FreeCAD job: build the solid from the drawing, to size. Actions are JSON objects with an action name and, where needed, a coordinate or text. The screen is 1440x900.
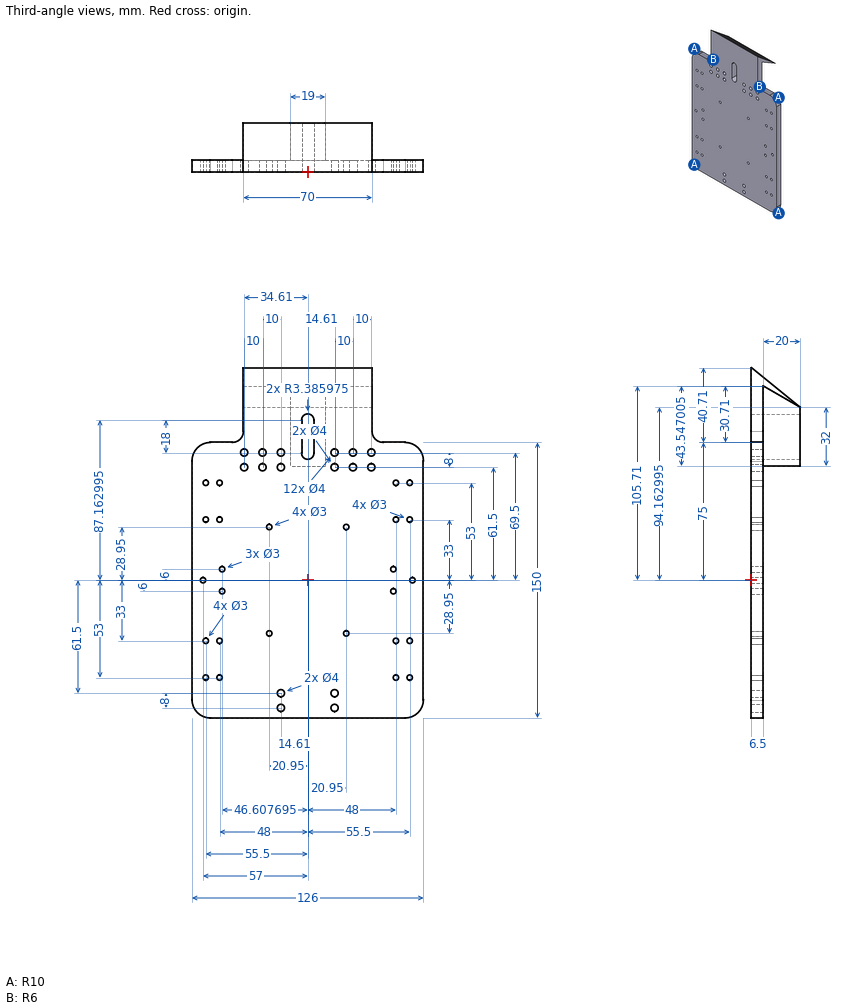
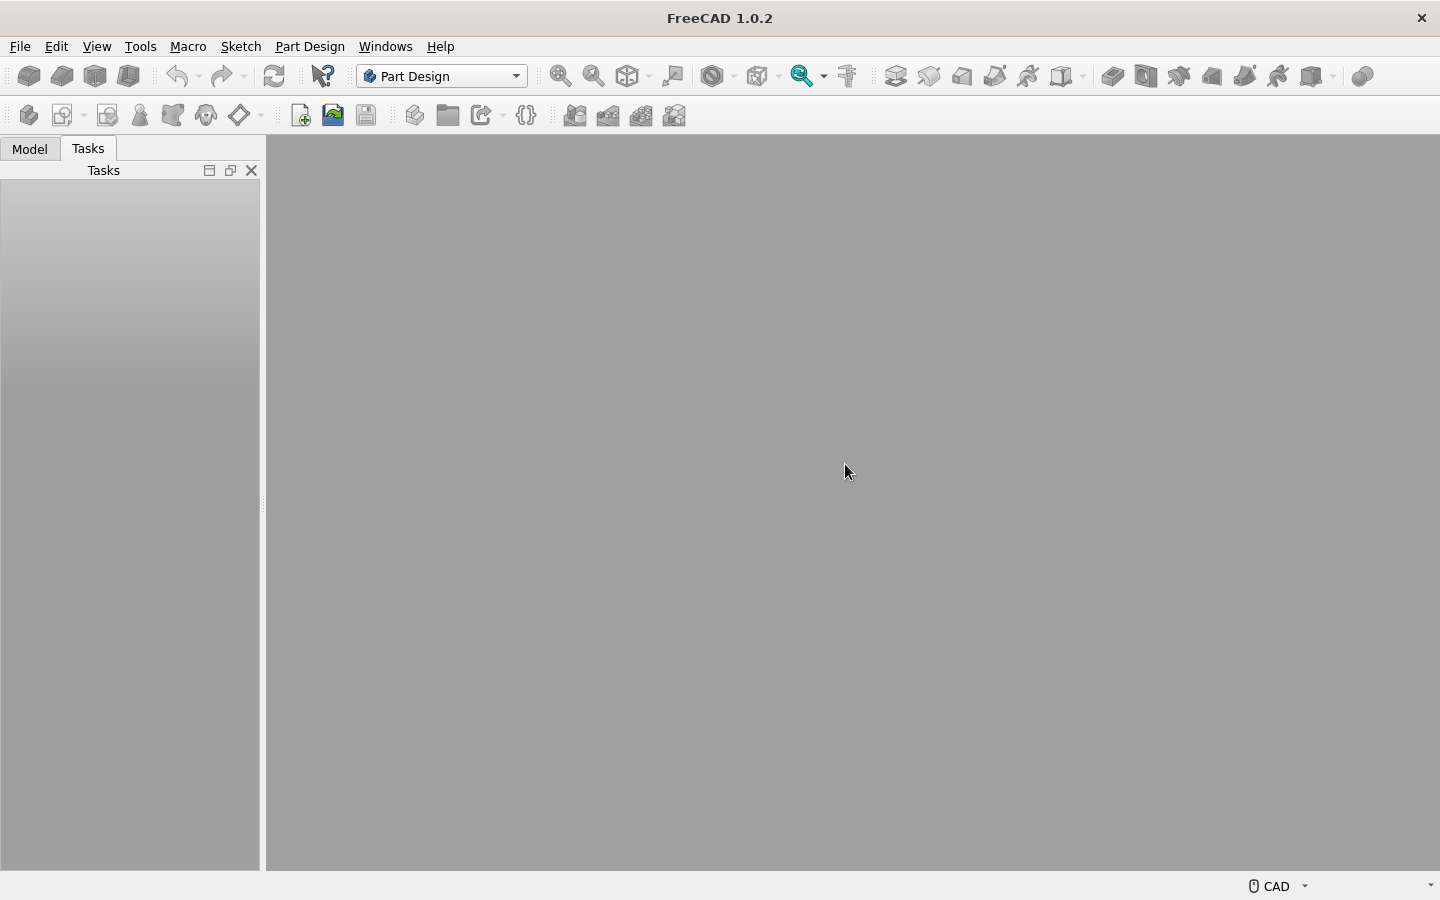
{"action": "left_click", "coordinate": [300, 116]}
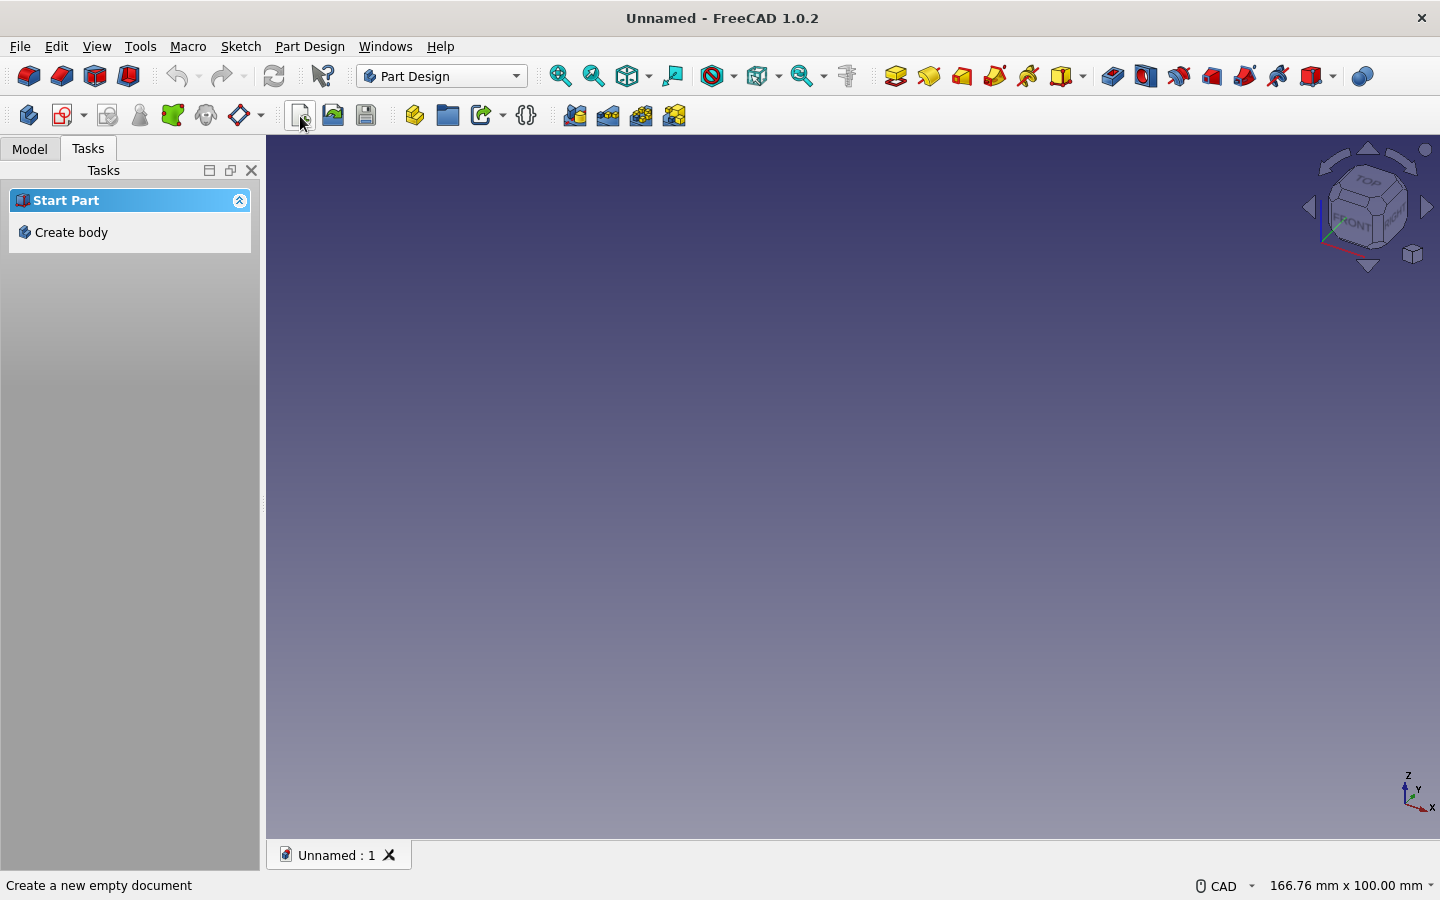
{"action": "left_click", "coordinate": [62, 116]}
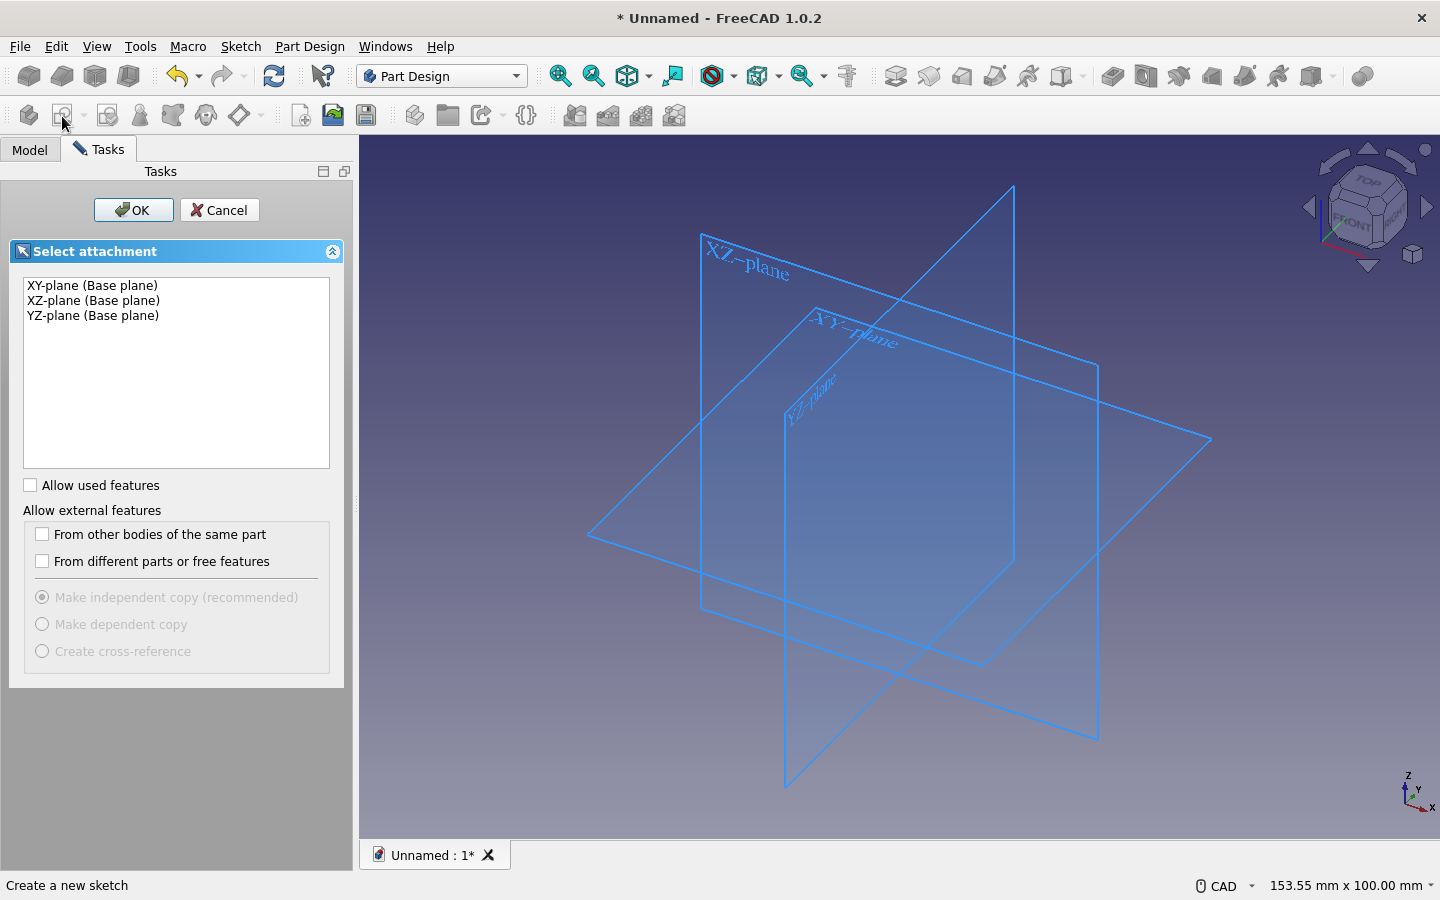
{"action": "left_click", "coordinate": [84, 300]}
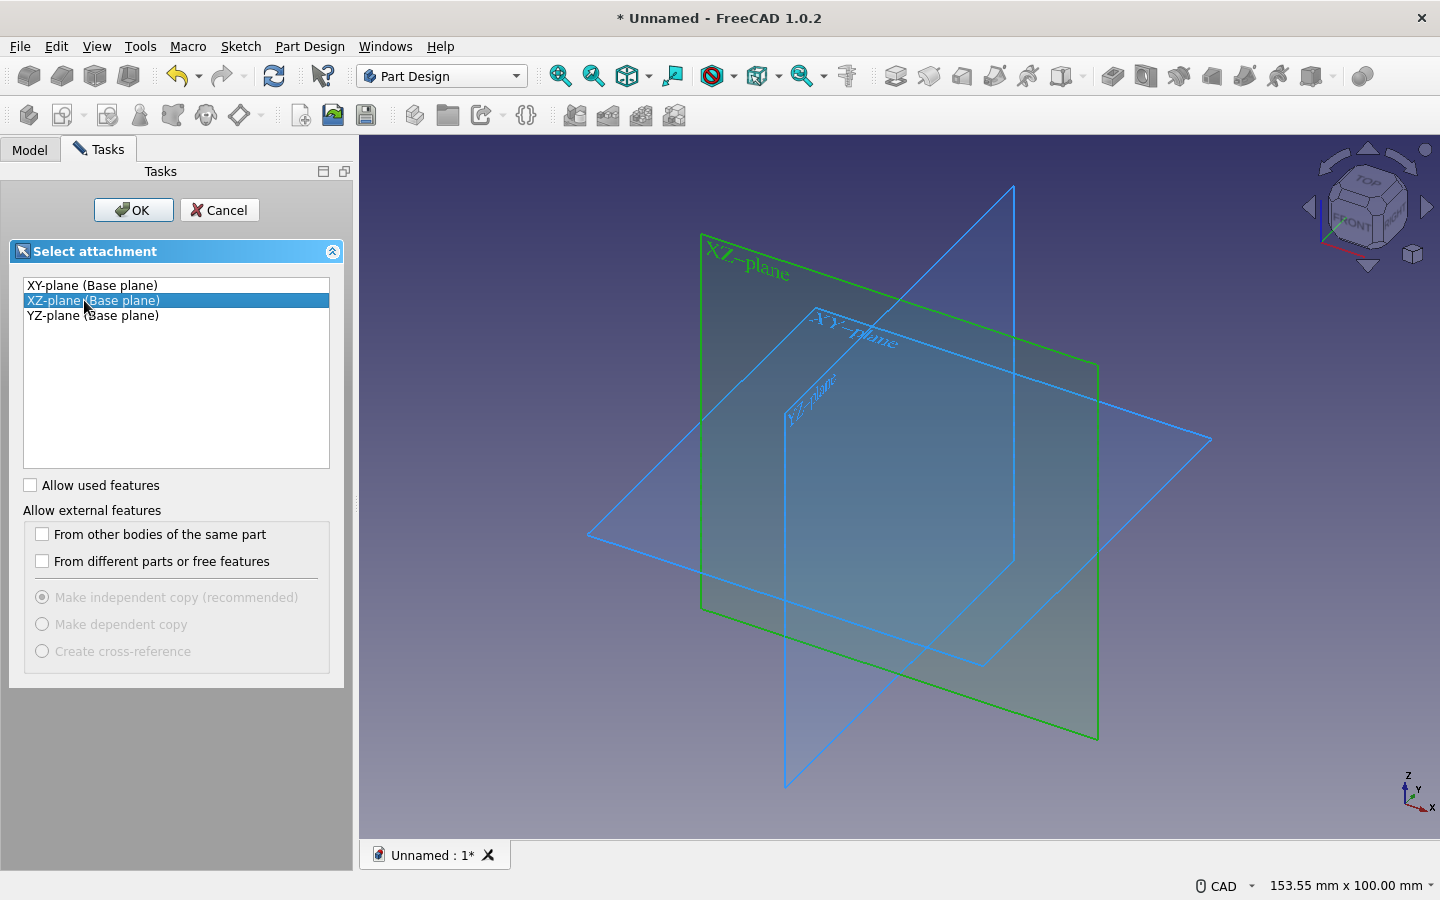
{"action": "left_click", "coordinate": [134, 210]}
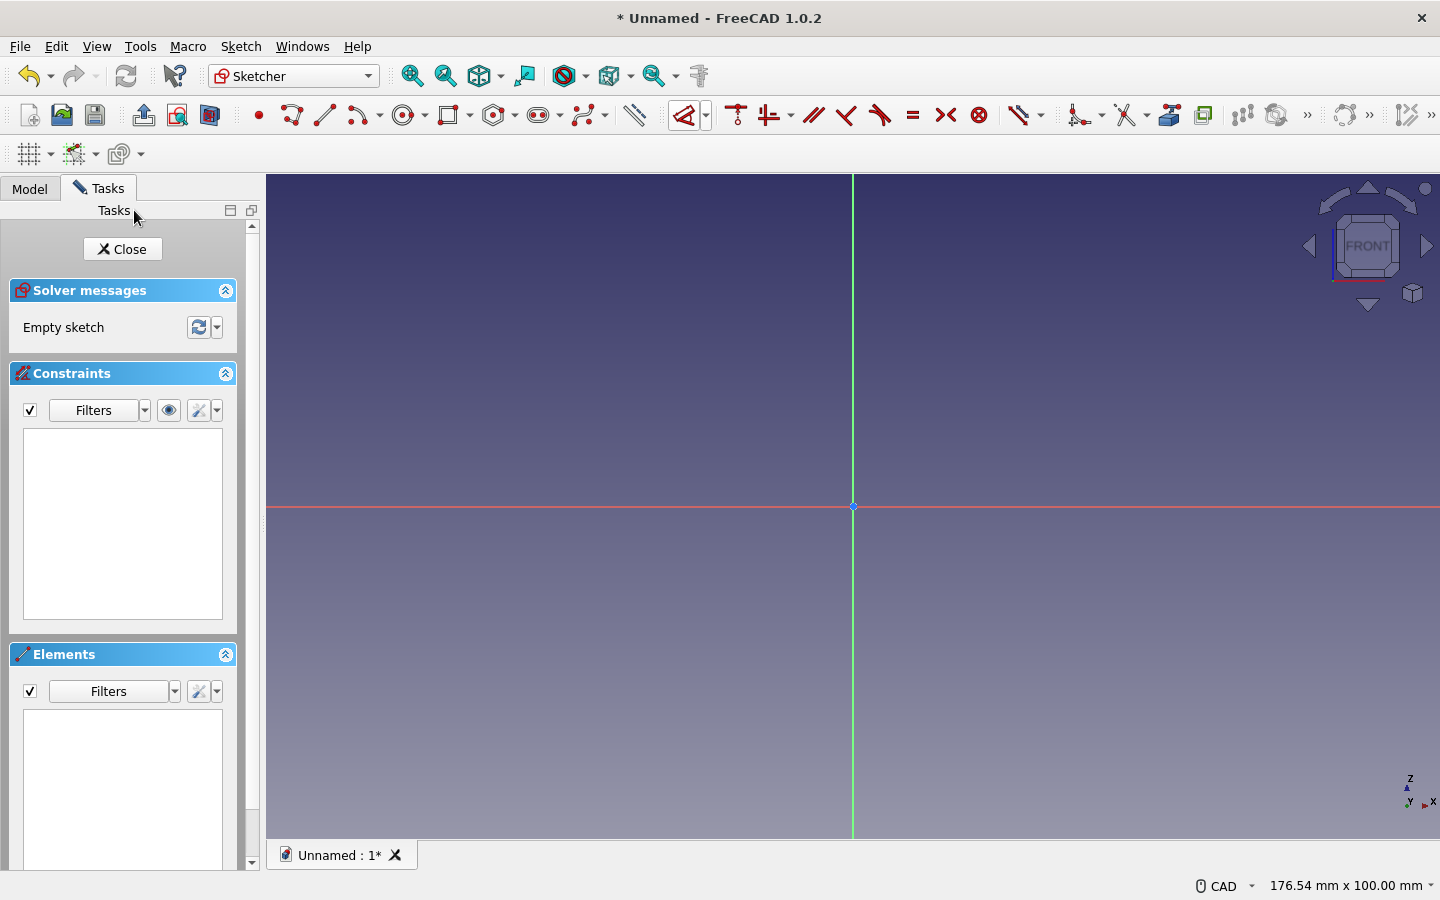
{"action": "scroll", "coordinate": [729, 506], "scroll_direction": "down", "scroll_amount": 4}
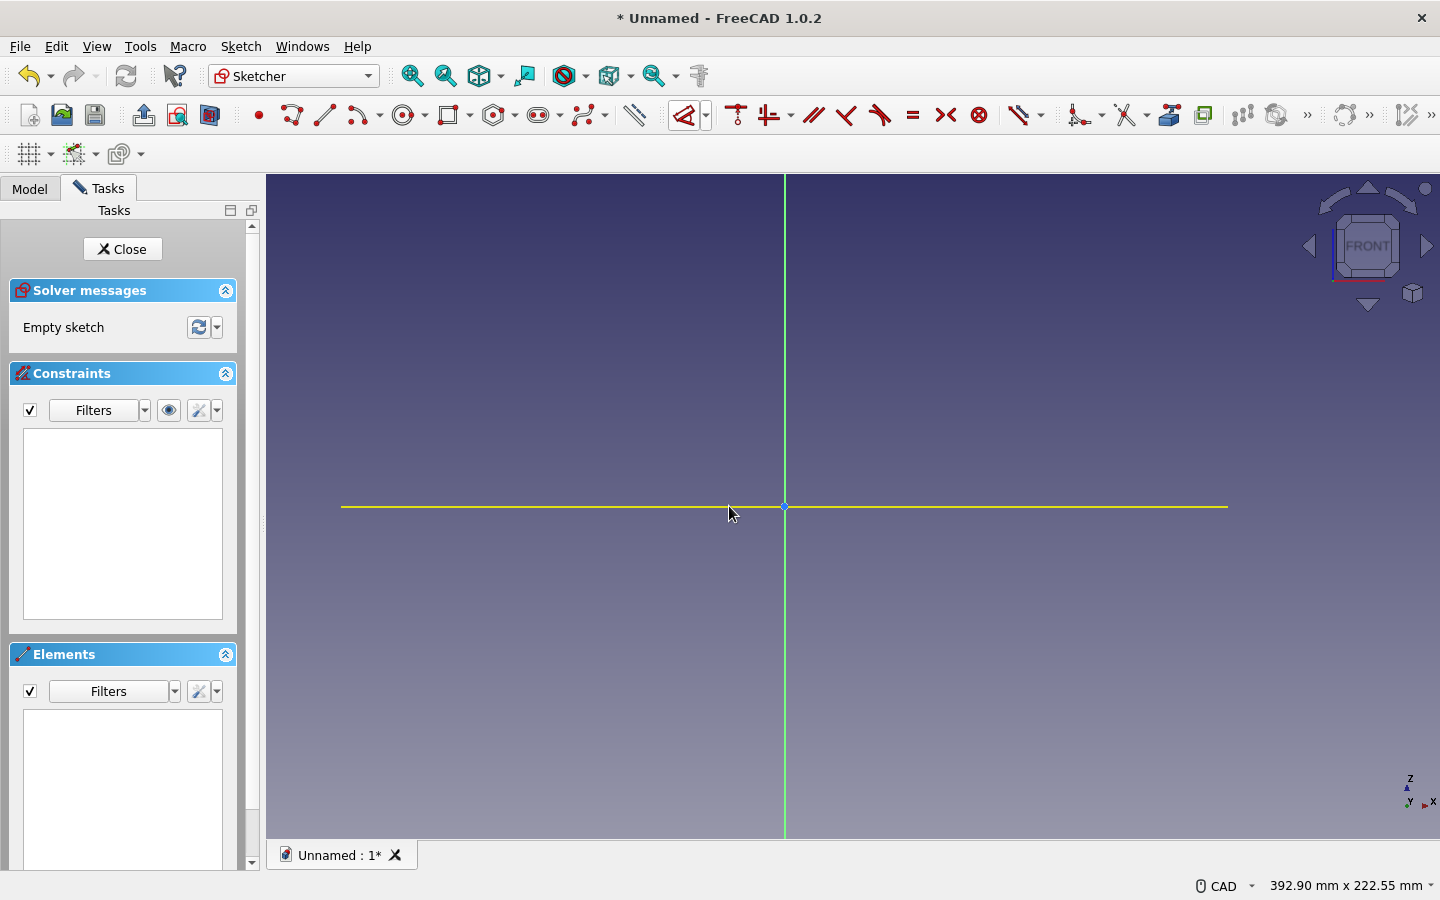
{"action": "key", "text": "g v"}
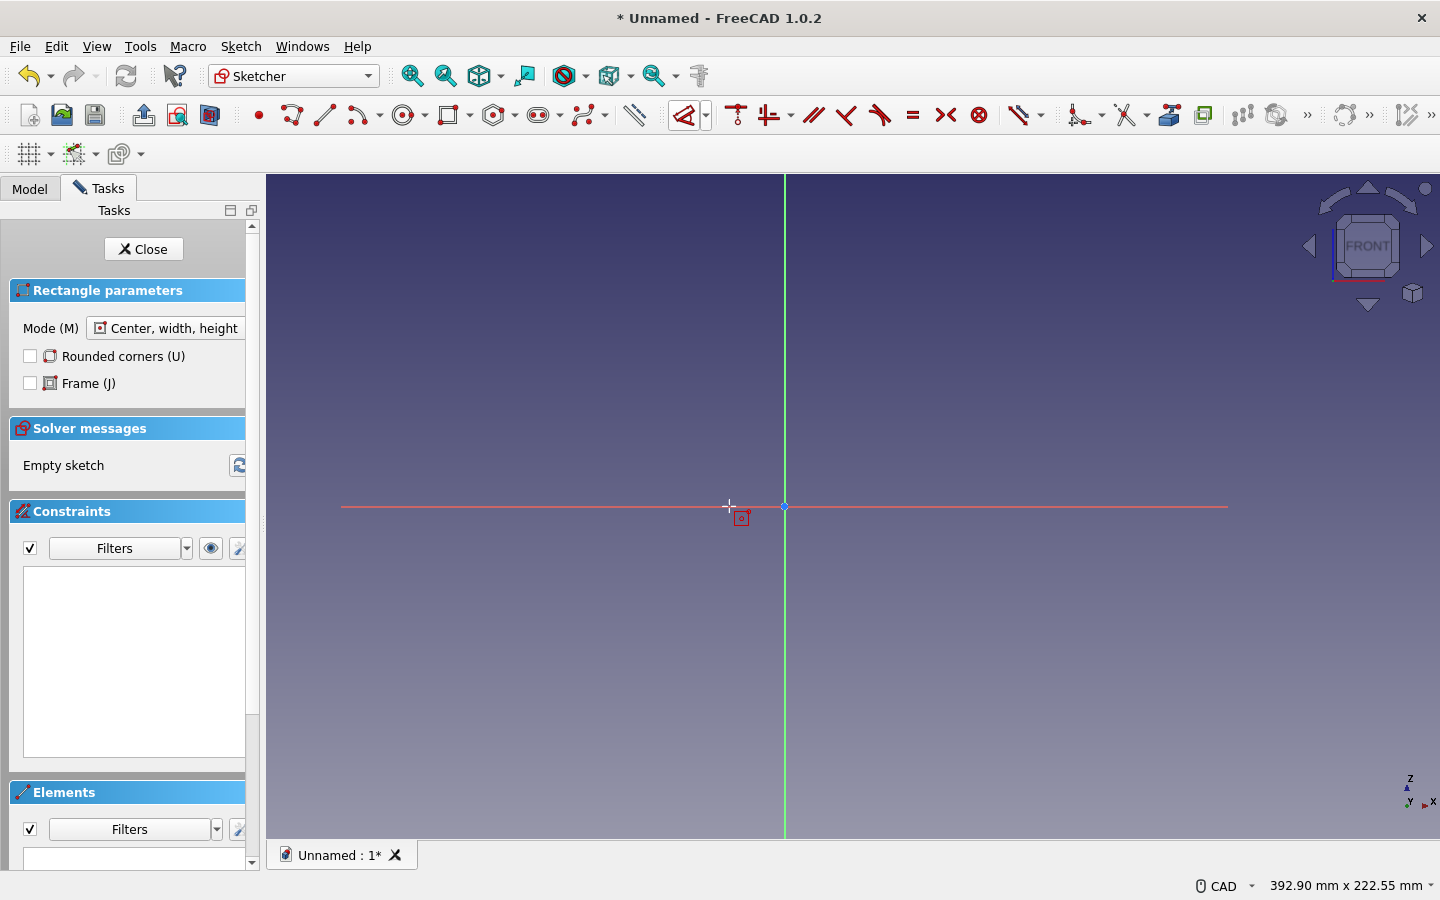
{"action": "left_click", "coordinate": [785, 506]}
{"action": "mouse_move", "coordinate": [973, 282]}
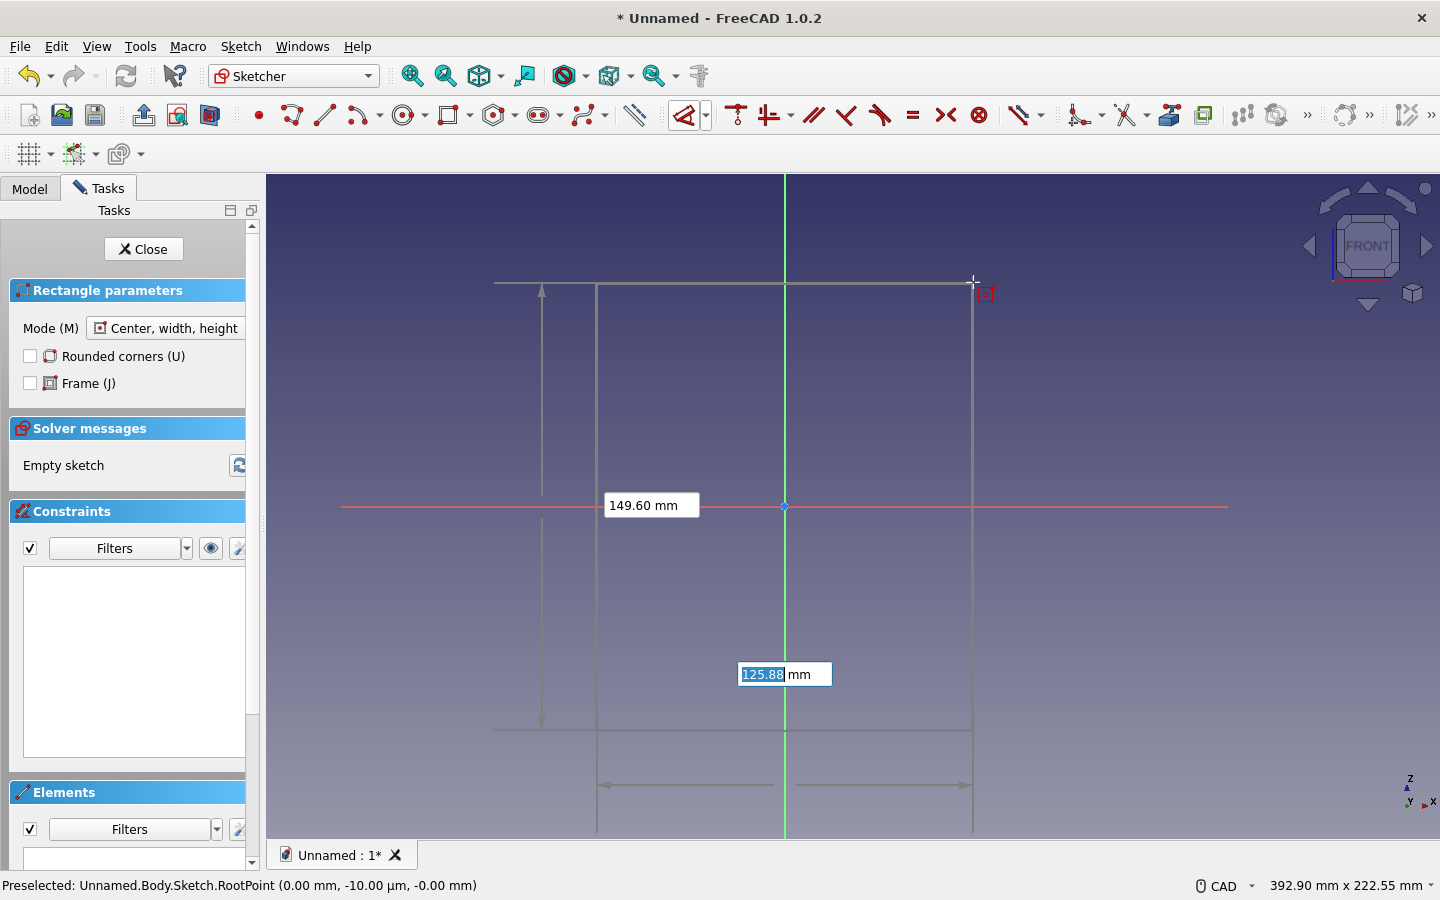
{"action": "type", "text": "126"}
{"action": "key", "text": "Tab"}
{"action": "type", "text": "150"}
{"action": "key", "text": "Return"}
{"action": "key", "text": "Escape"}